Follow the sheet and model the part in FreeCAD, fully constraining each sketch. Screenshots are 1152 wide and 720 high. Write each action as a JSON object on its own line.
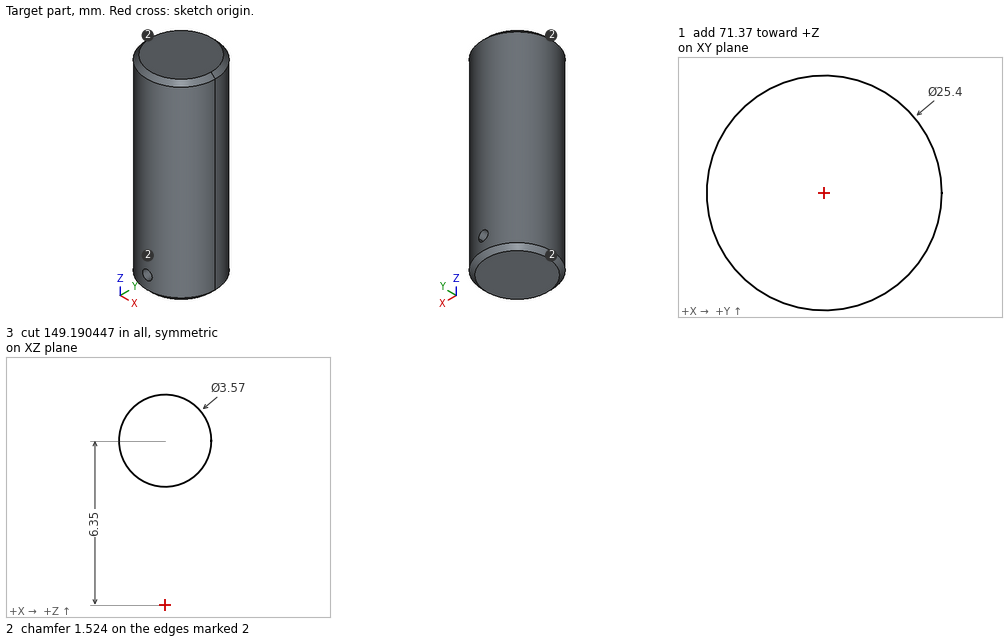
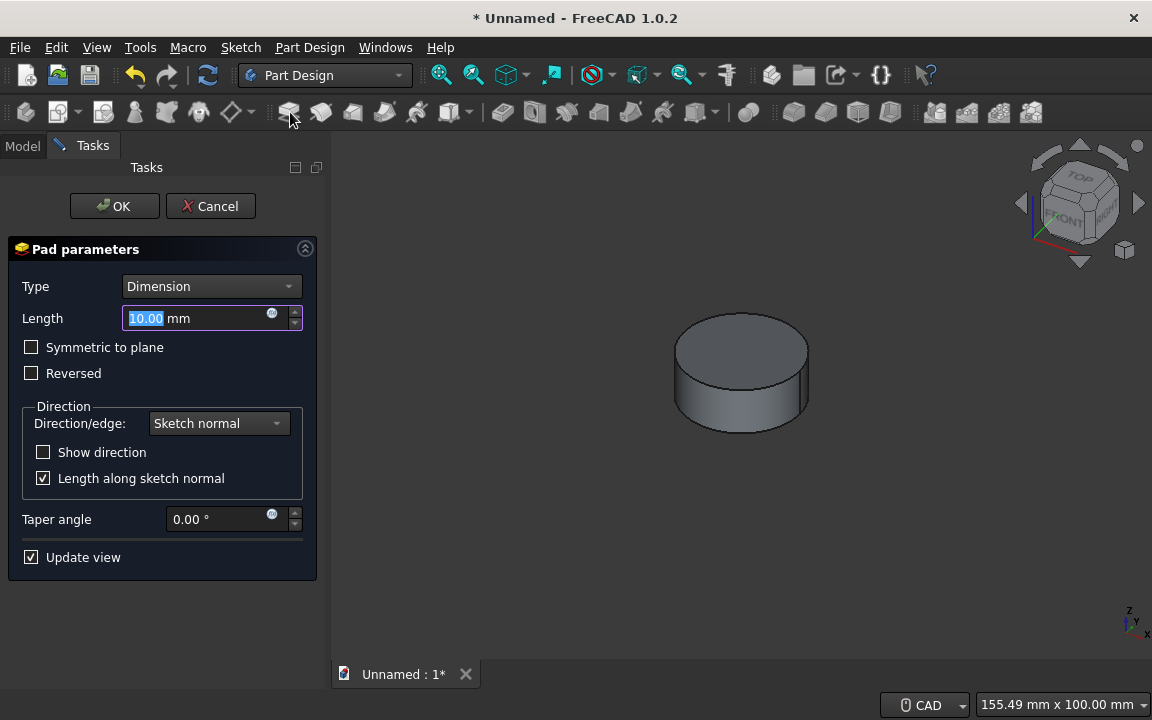
{"action": "type", "text": "71.37"}
{"action": "key", "text": "Tab"}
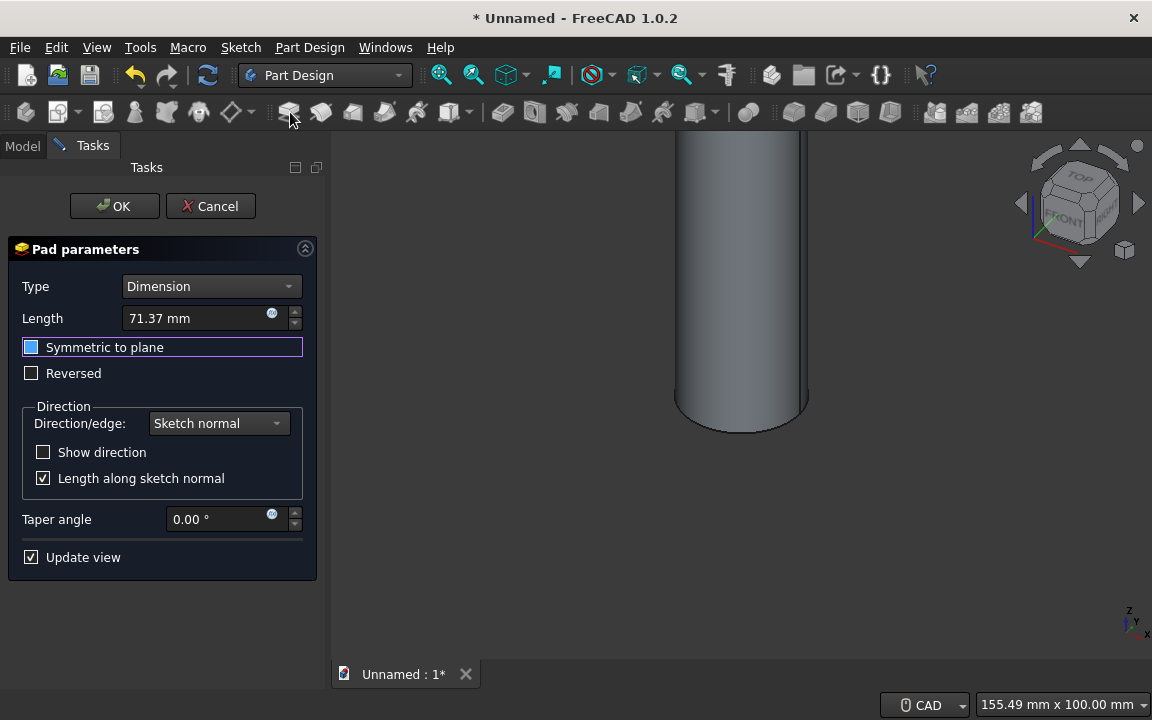
{"action": "left_click", "coordinate": [115, 206]}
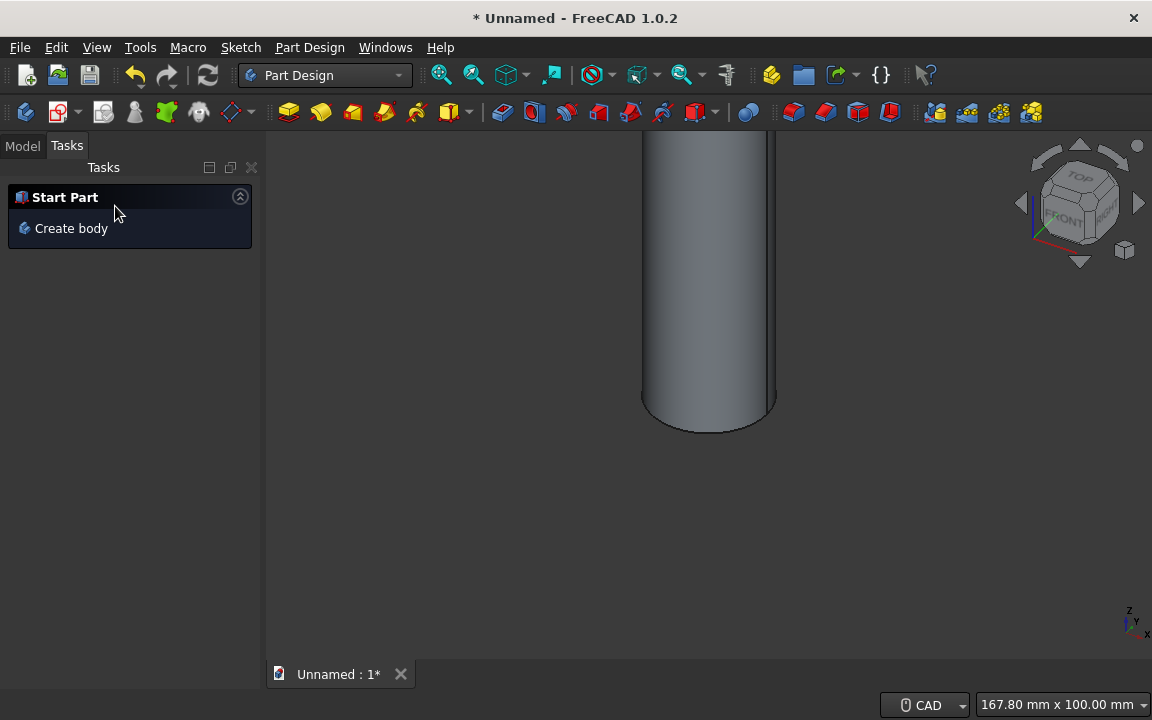
{"action": "left_click", "coordinate": [442, 76]}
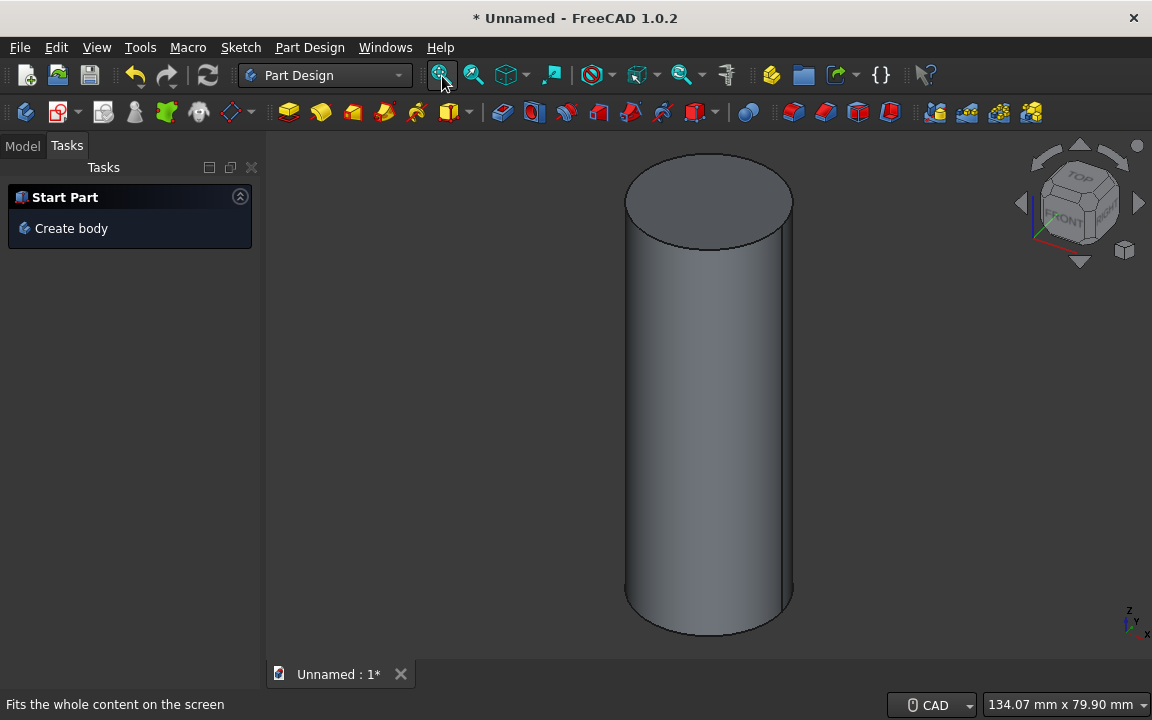
{"action": "left_click", "coordinate": [626, 206]}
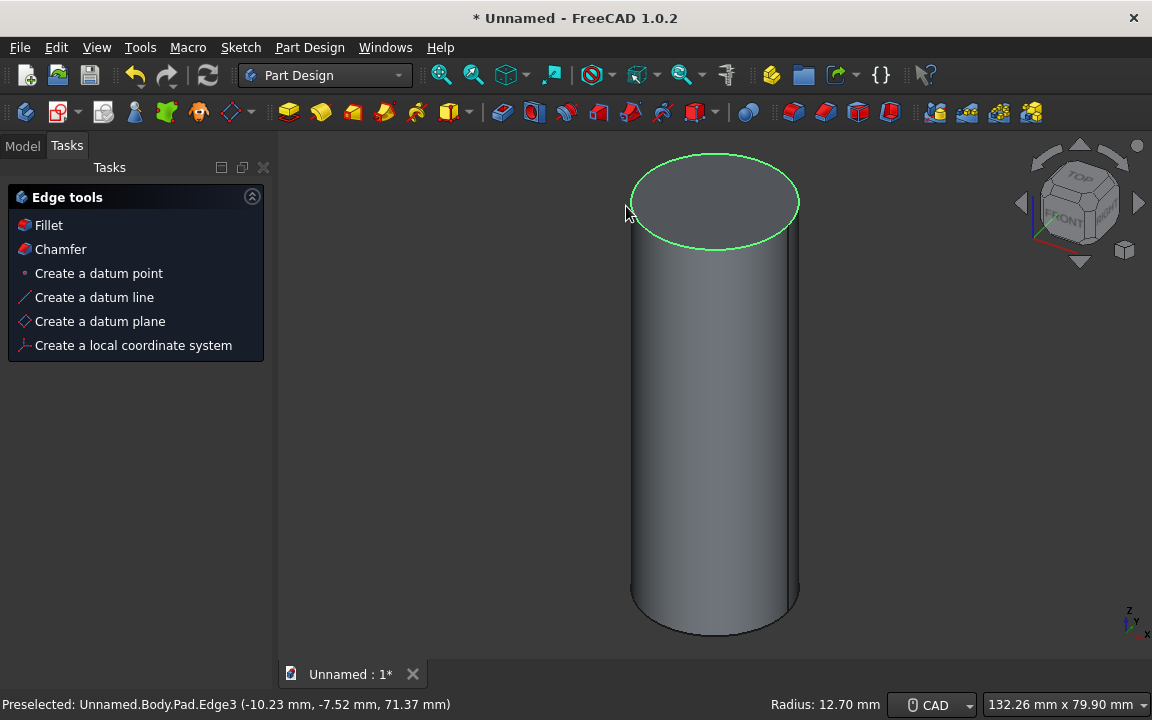
{"action": "key", "text": "0"}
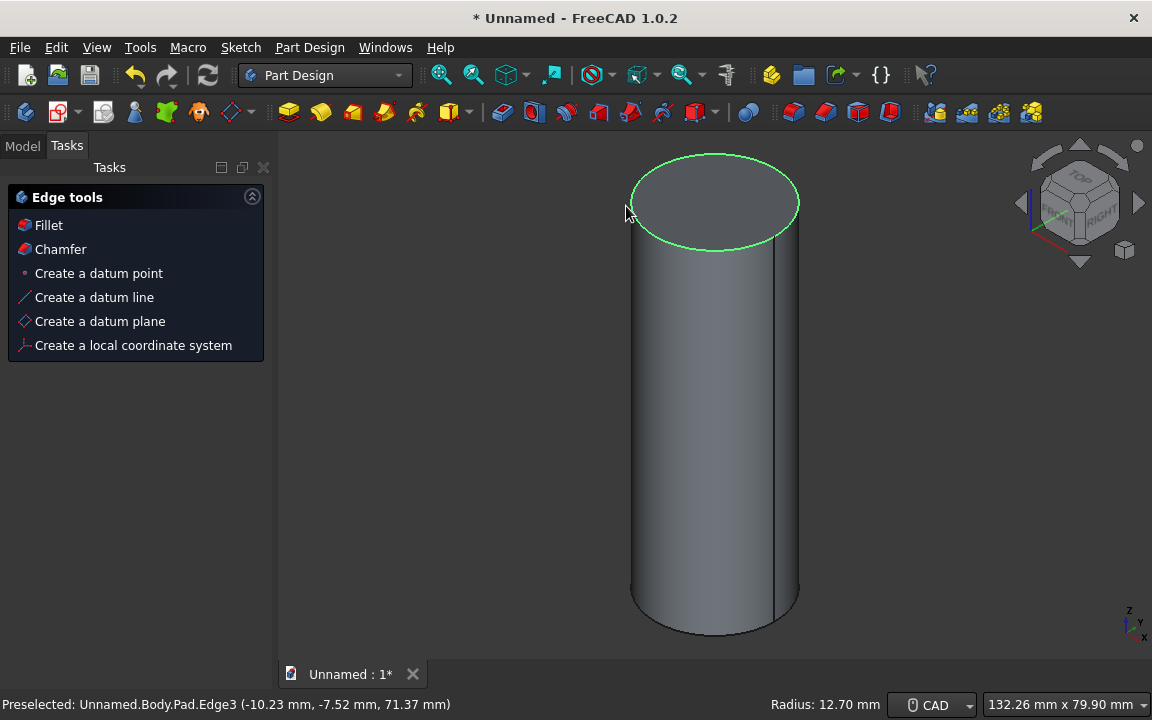
{"action": "key", "text": "2"}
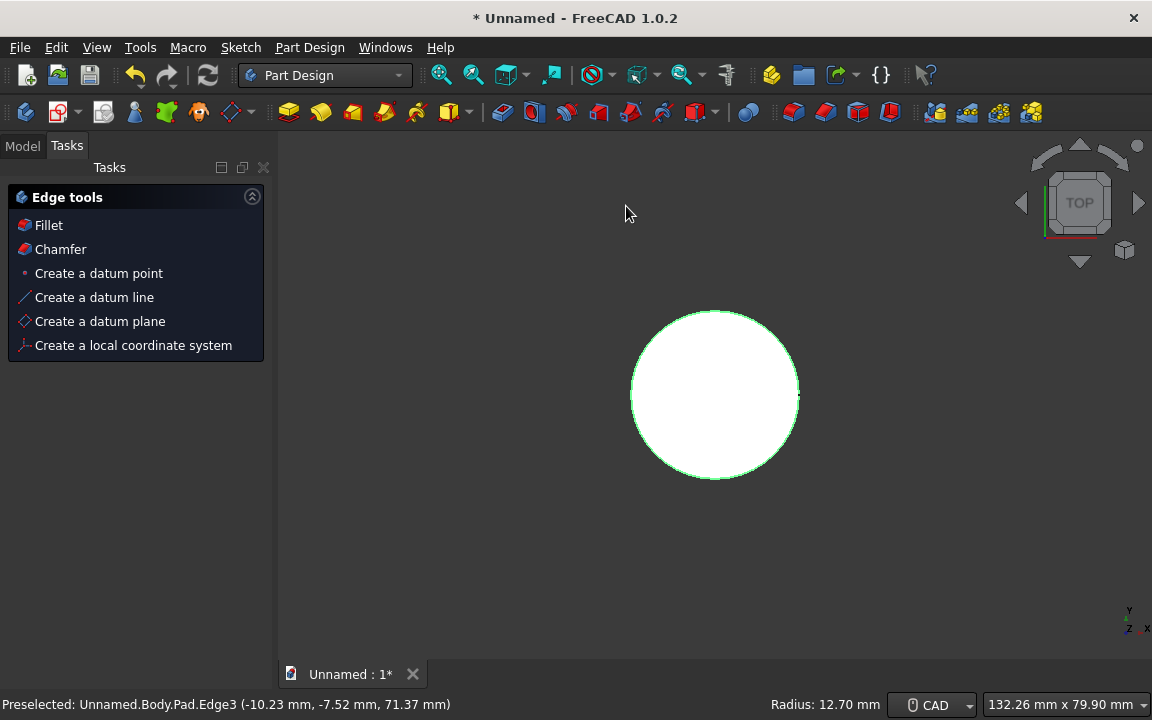
{"action": "left_click", "coordinate": [442, 76]}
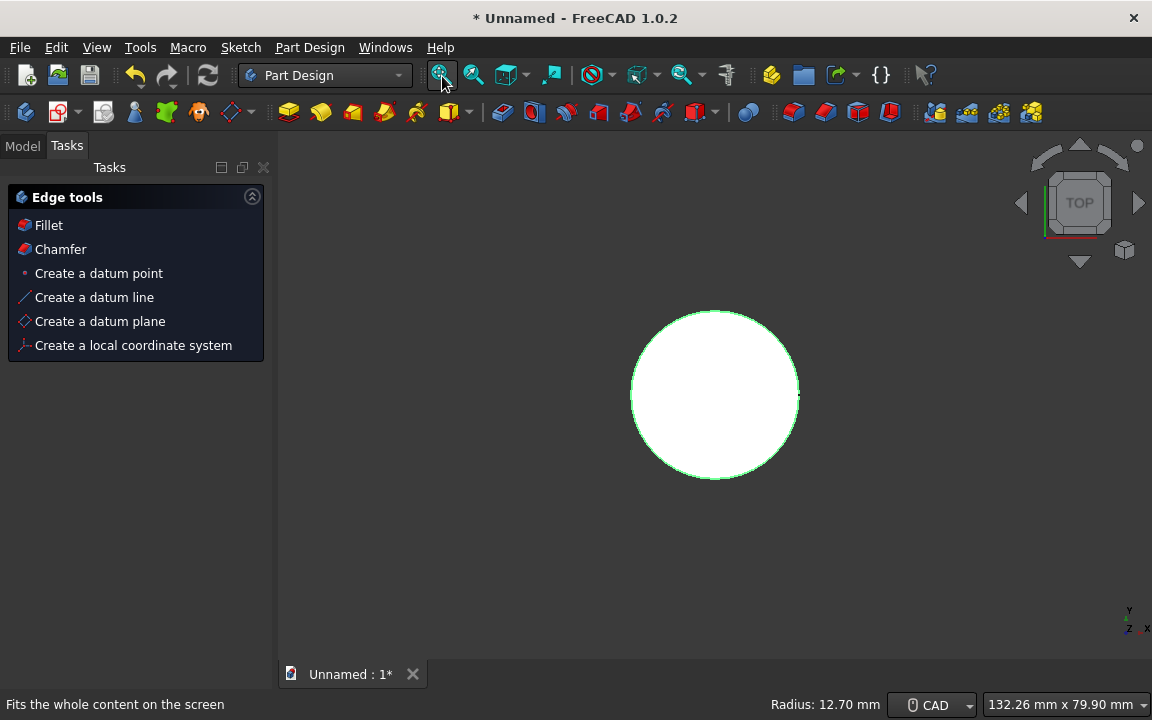
{"action": "key", "text": "1"}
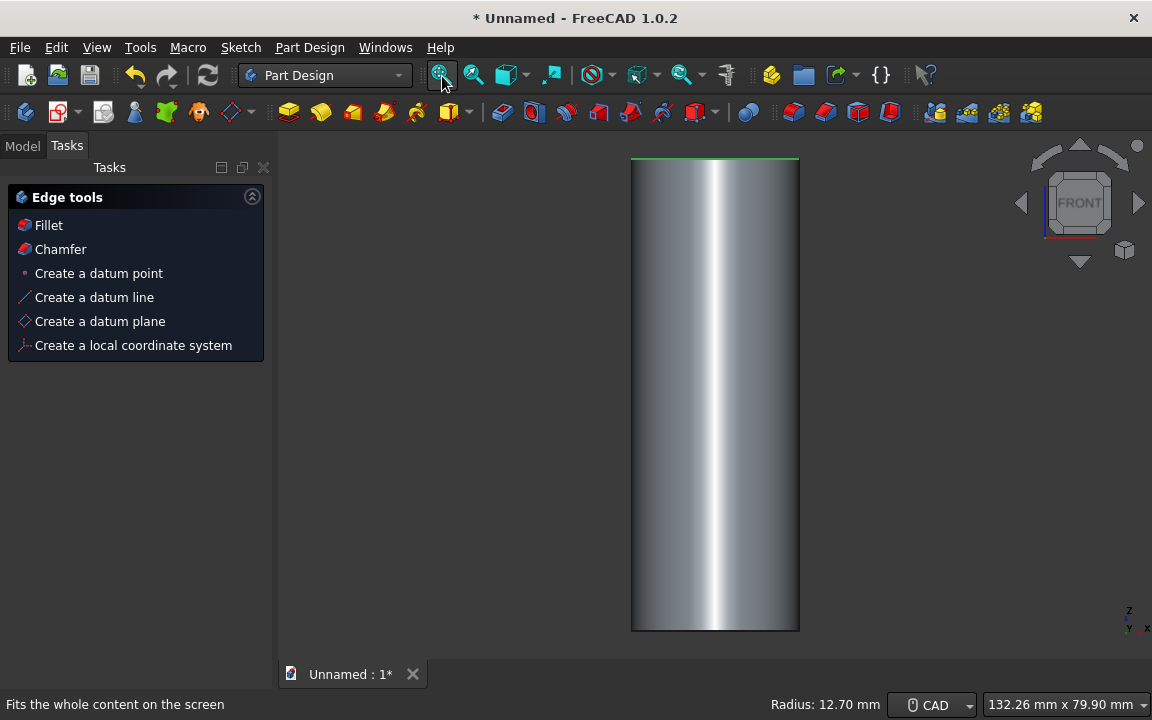
{"action": "left_click", "coordinate": [647, 630], "text": "ctrl"}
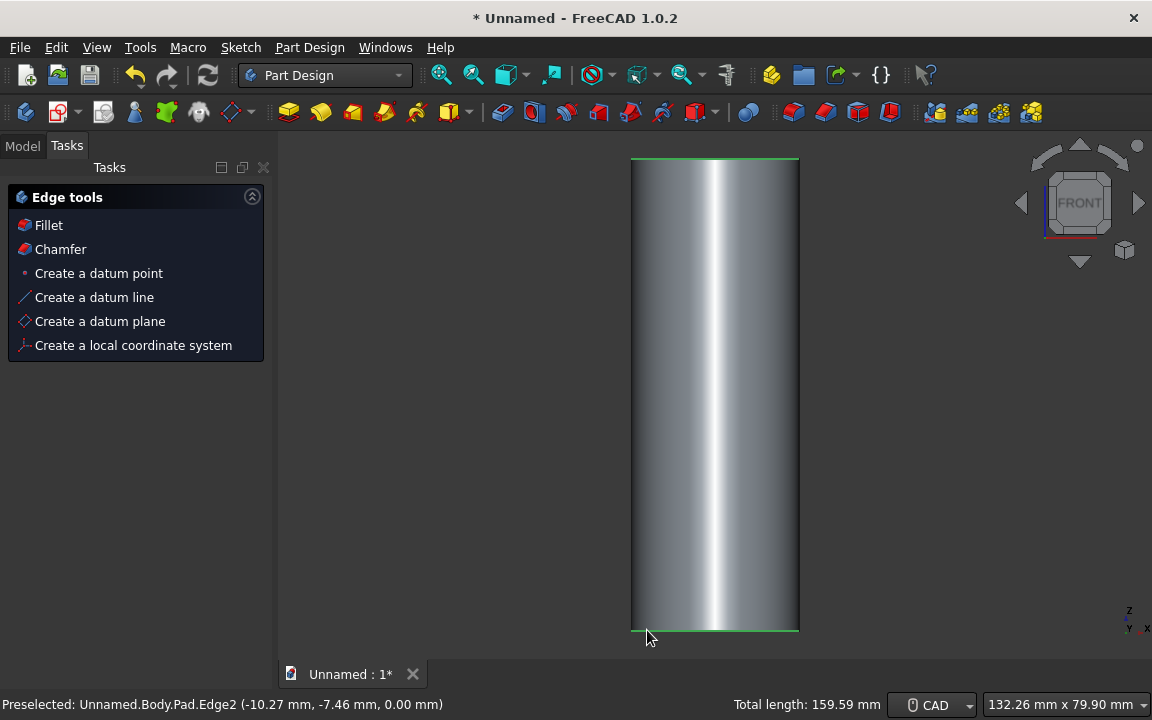
{"action": "left_click", "coordinate": [826, 112]}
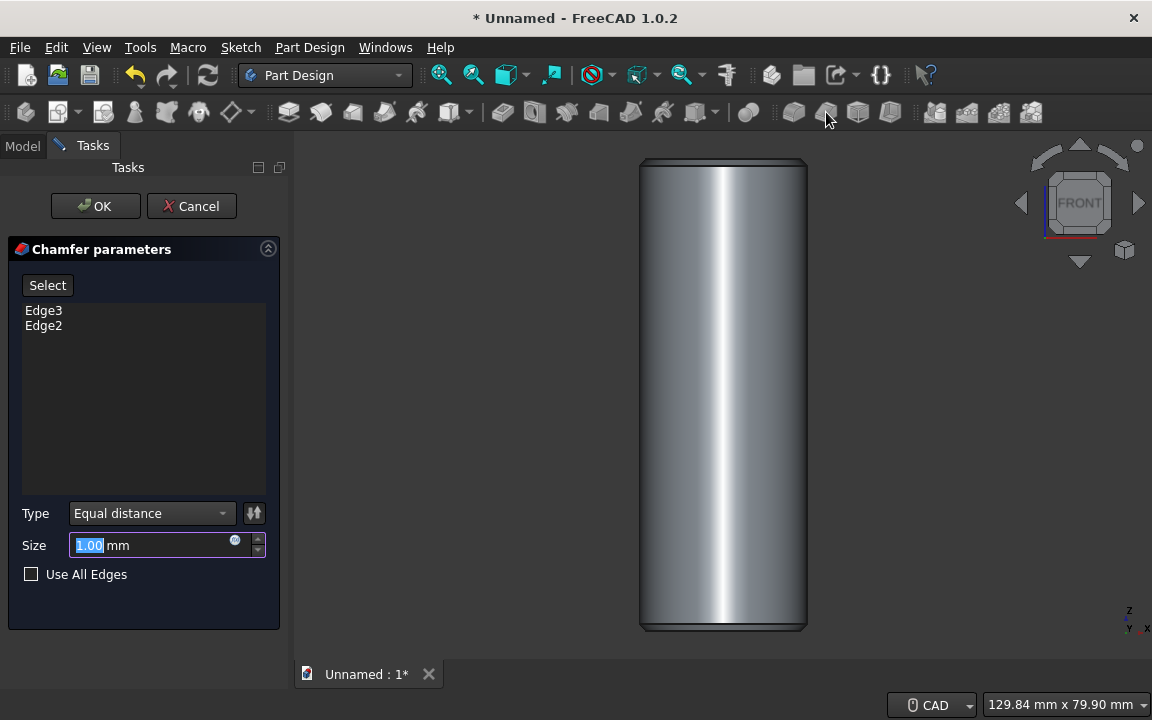
{"action": "type", "text": "1.524"}
{"action": "key", "text": "Tab"}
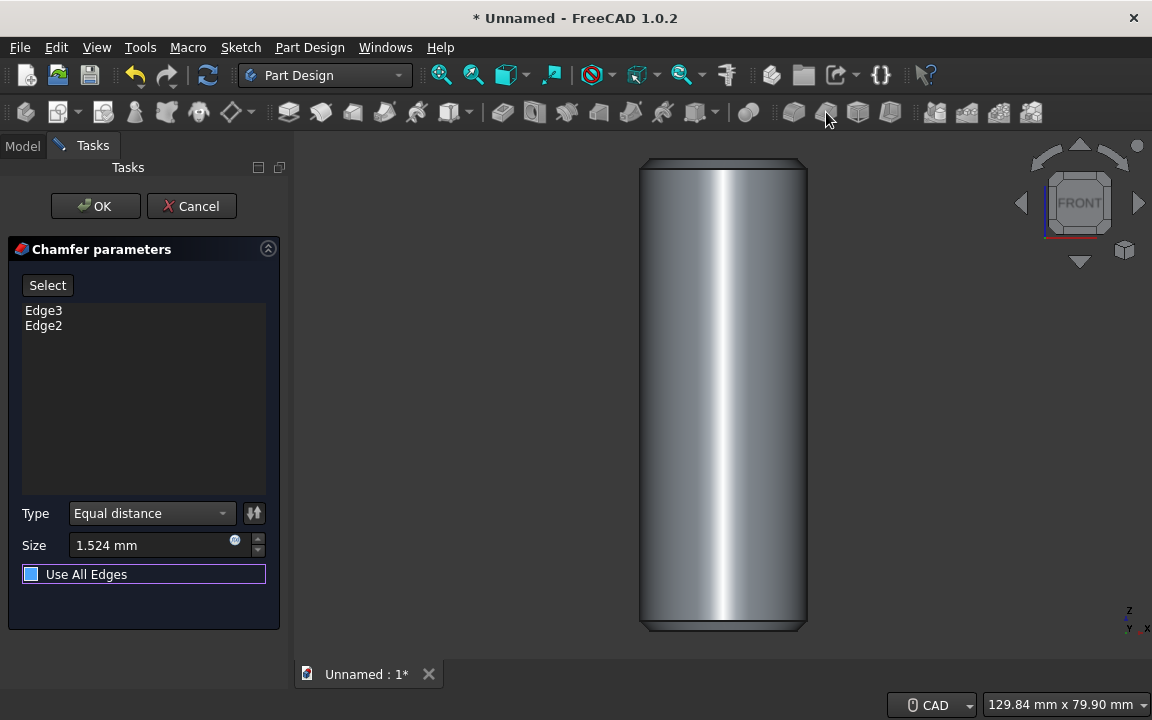
{"action": "left_click", "coordinate": [96, 206]}